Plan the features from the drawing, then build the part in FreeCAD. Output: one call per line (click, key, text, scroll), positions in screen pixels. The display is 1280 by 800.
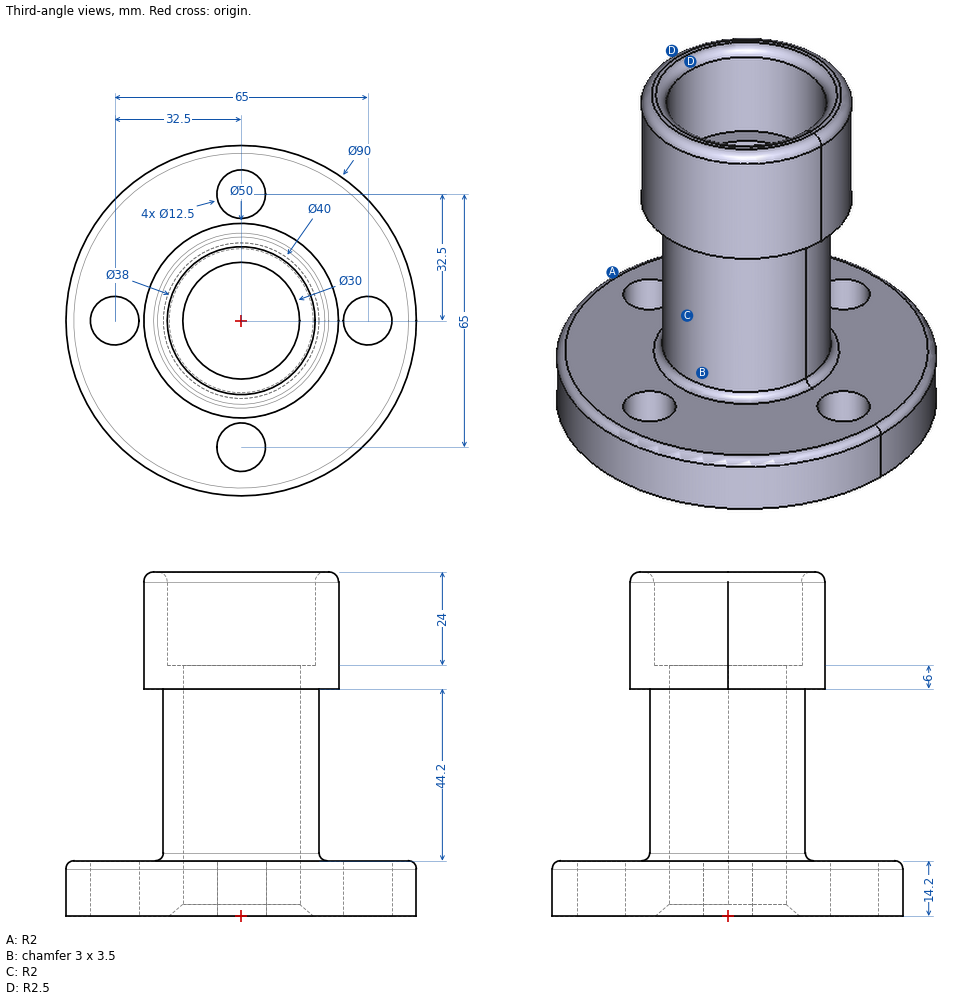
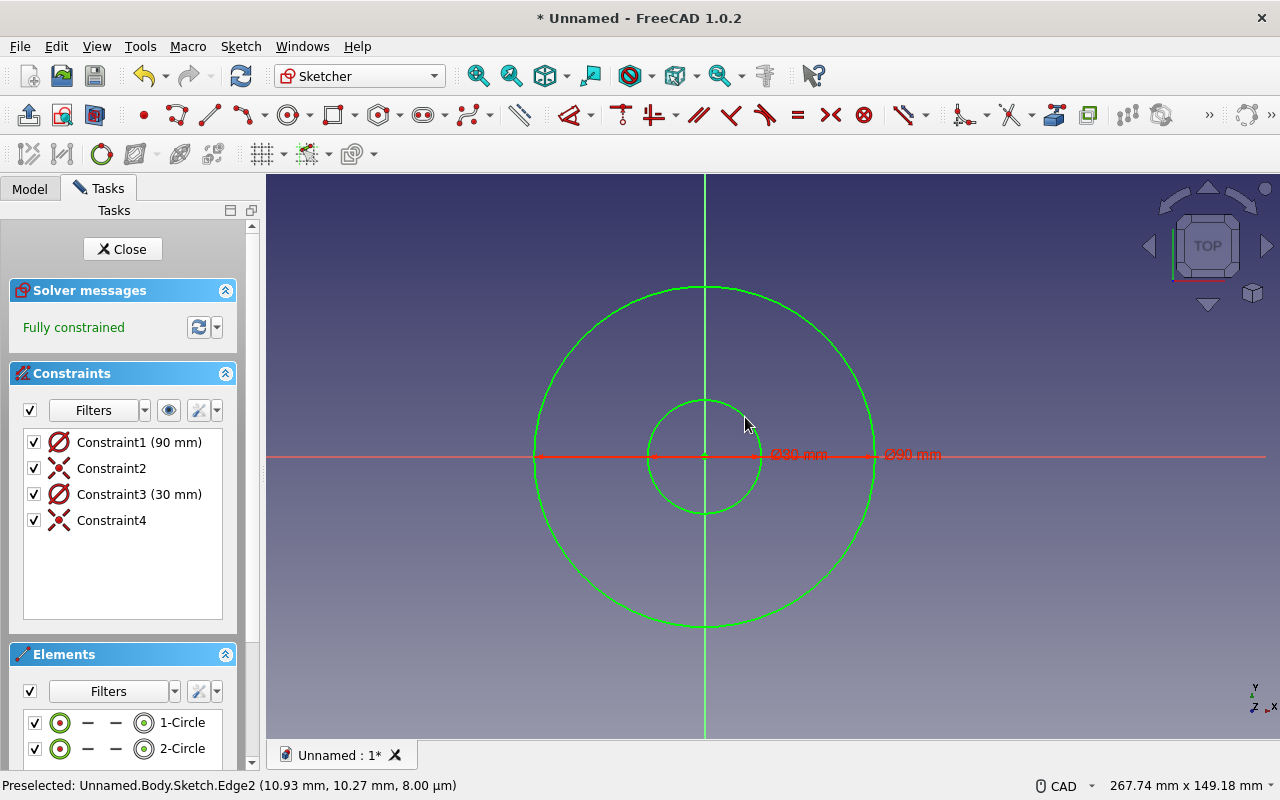
click(123, 249)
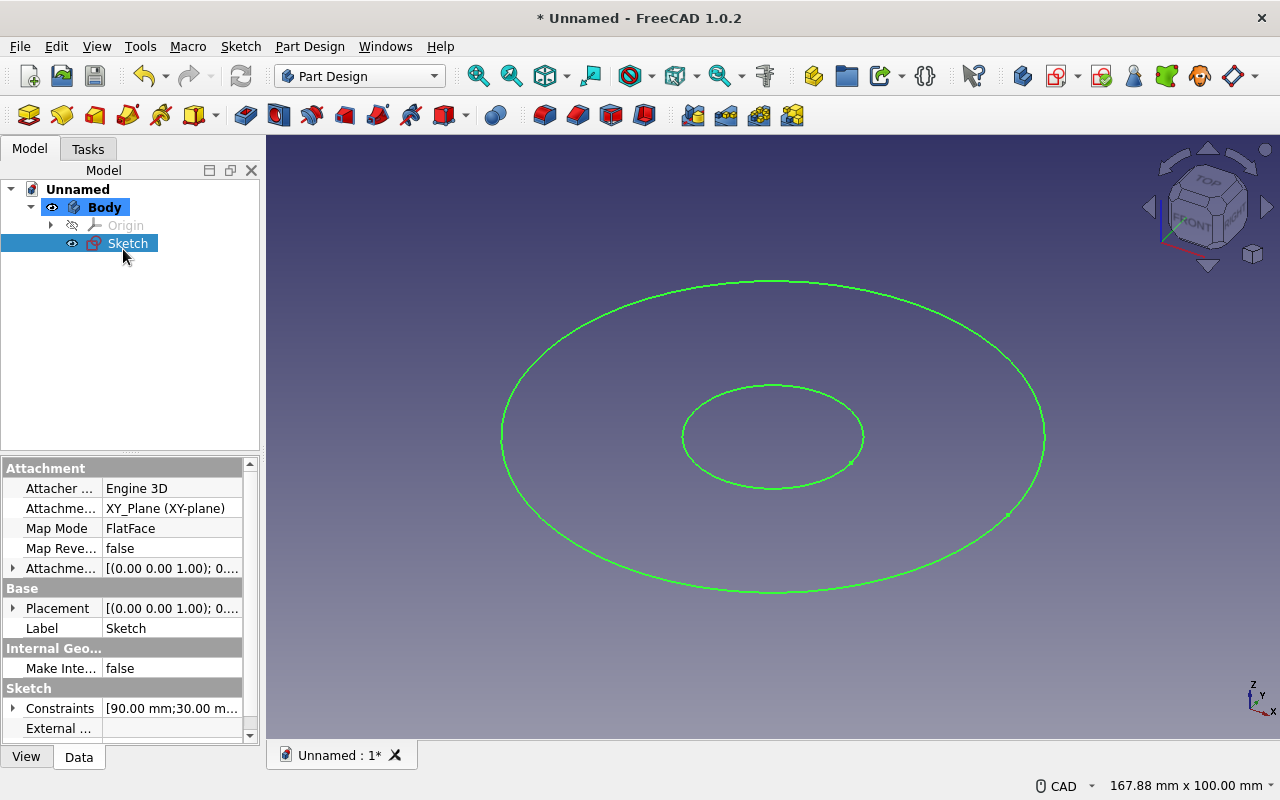
click(29, 116)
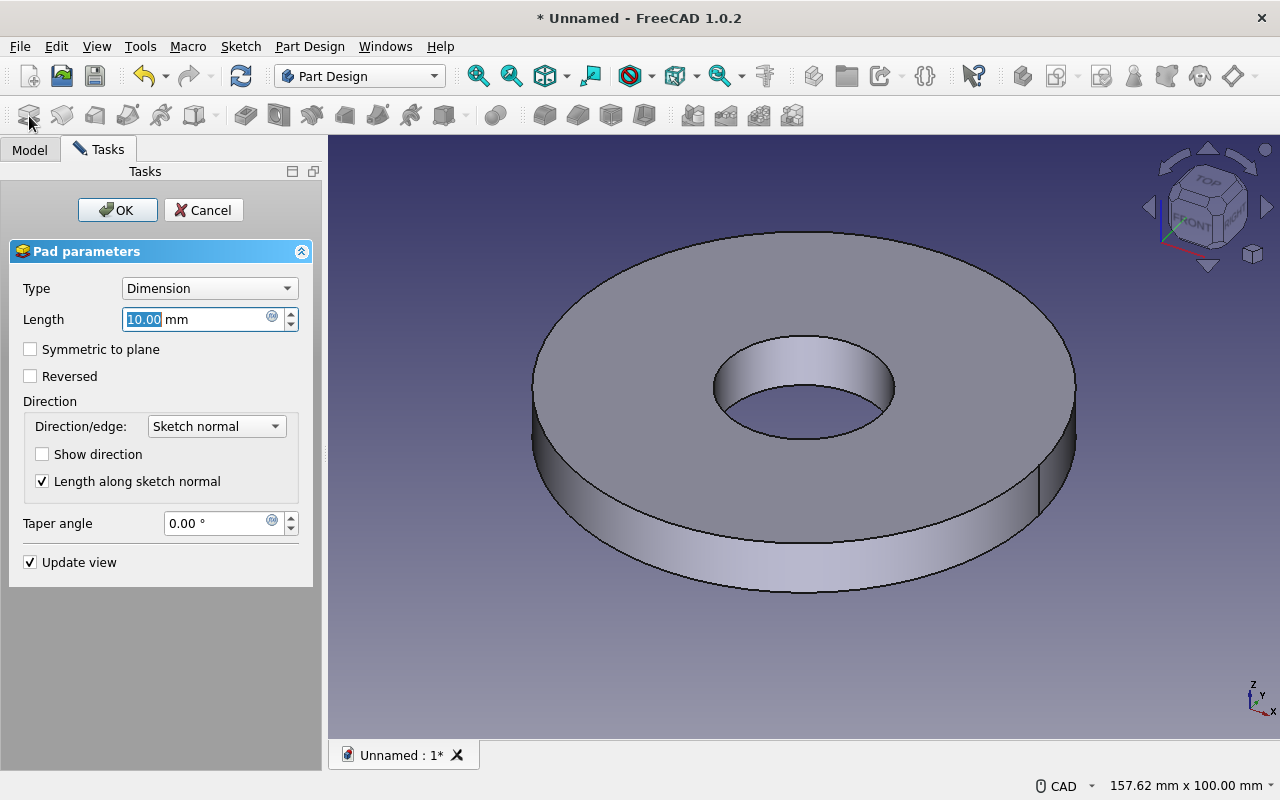
text(14.2)
key(Tab)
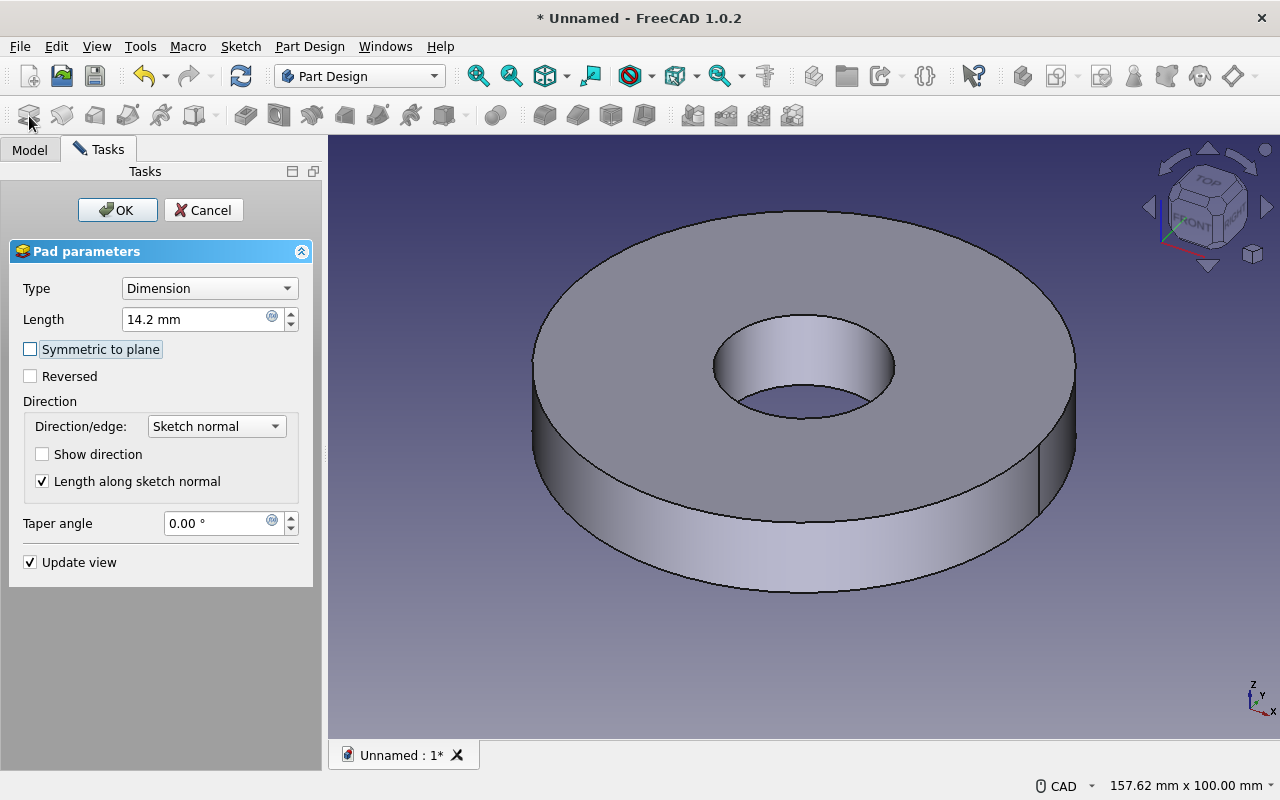
click(118, 210)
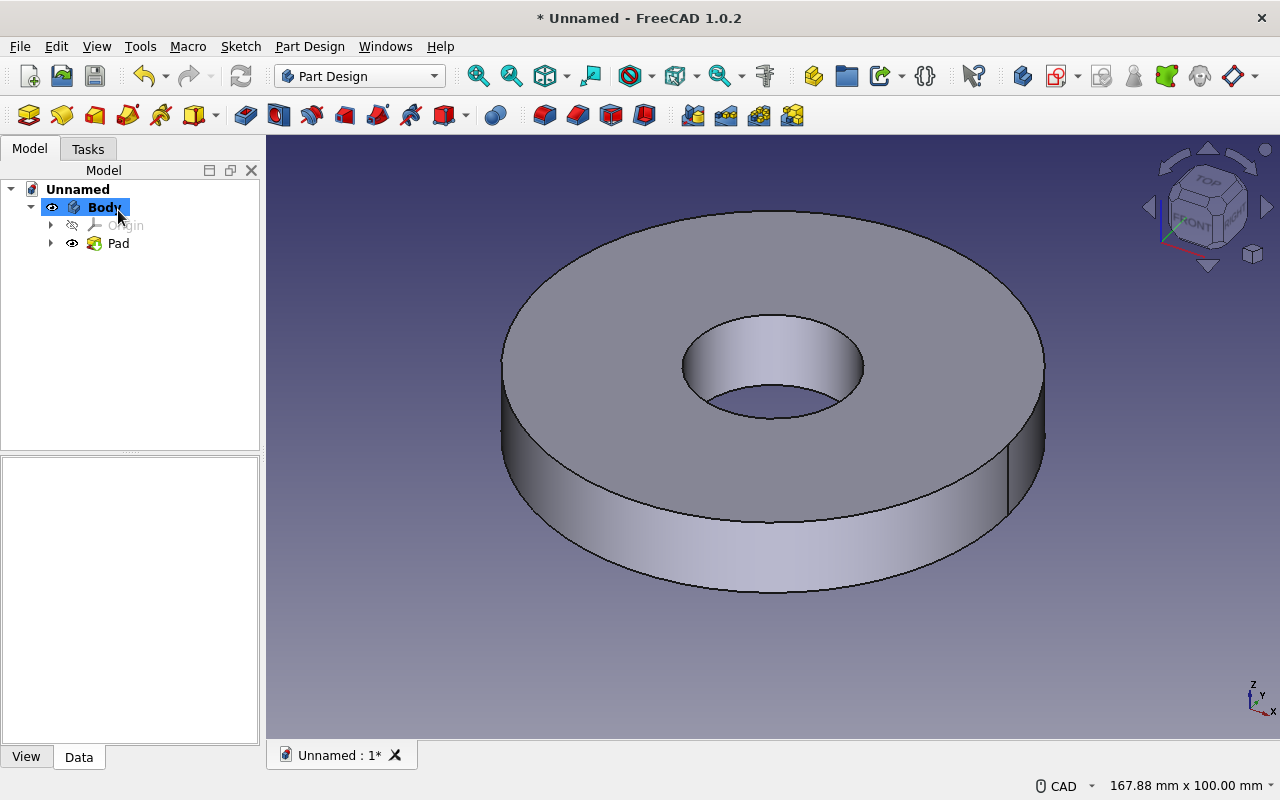
click(628, 421)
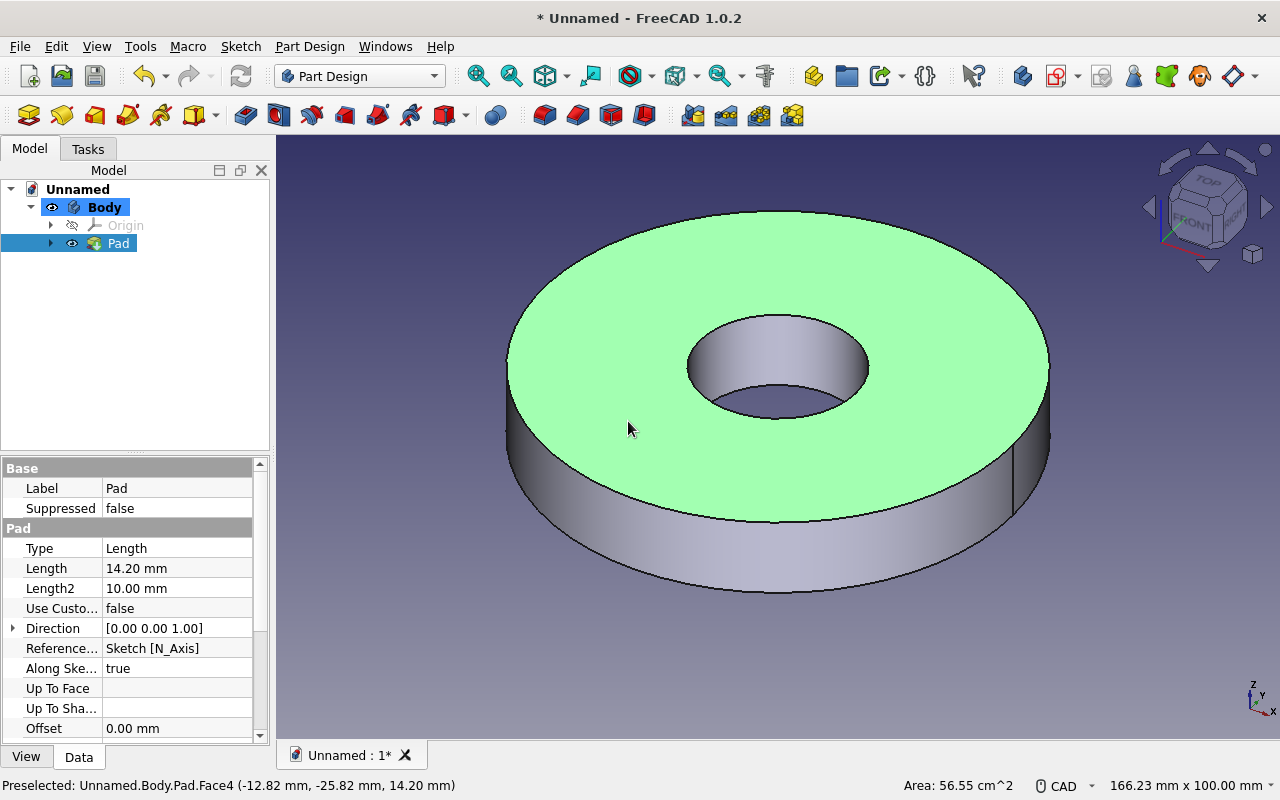
click(1056, 76)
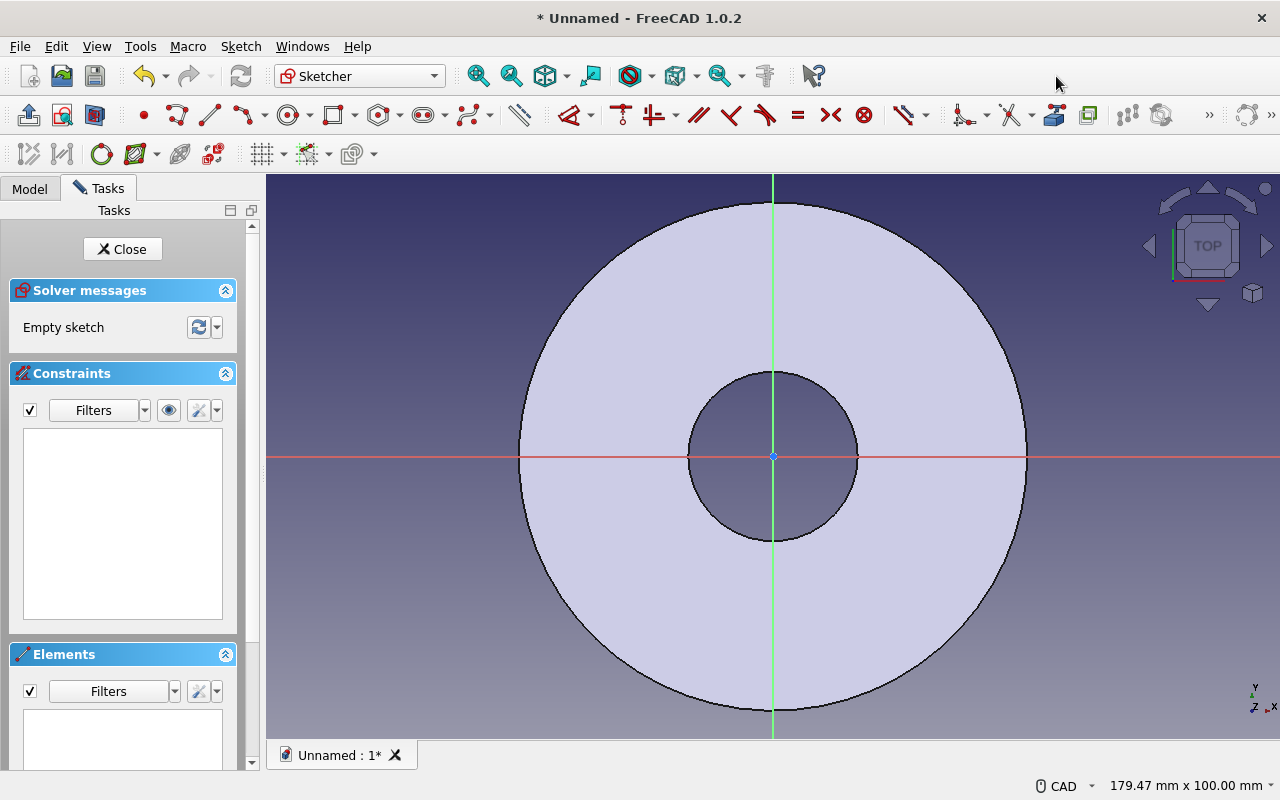
key(g)
key(c)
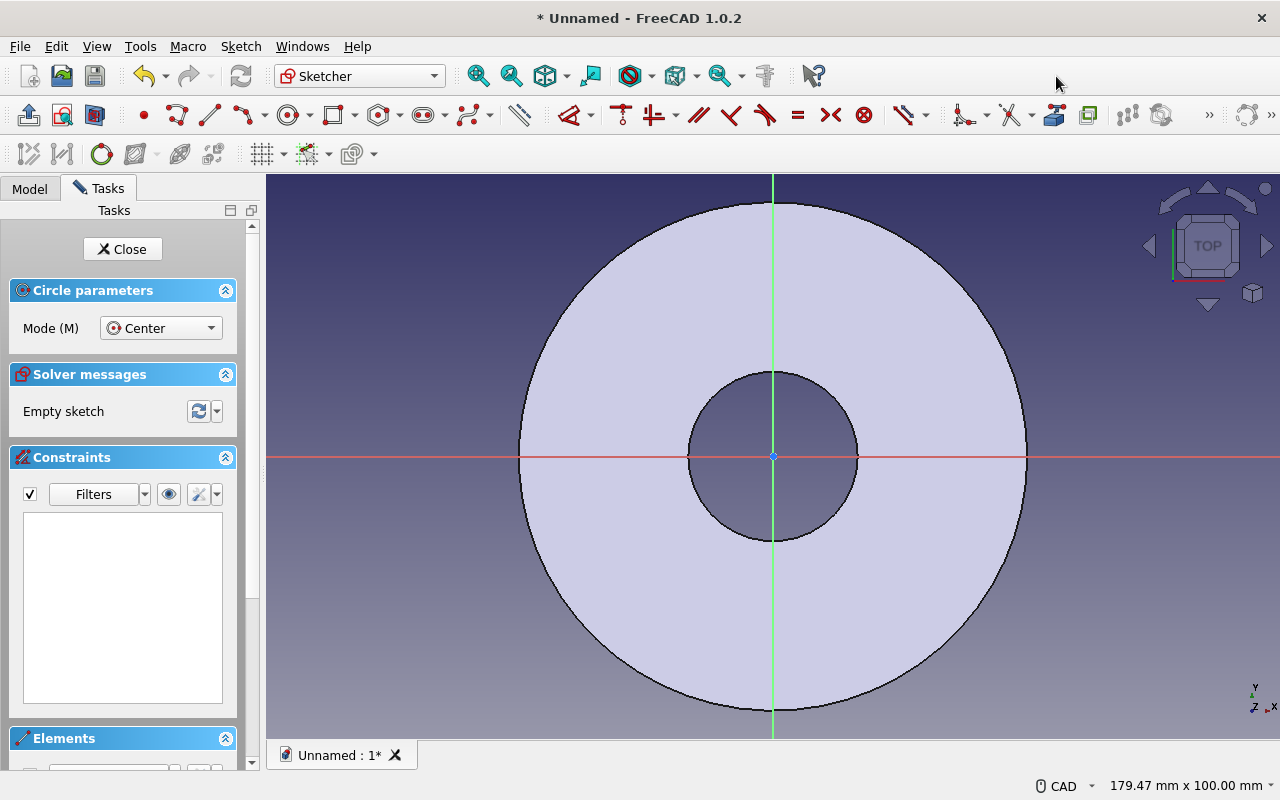
click(773, 273)
move(798, 248)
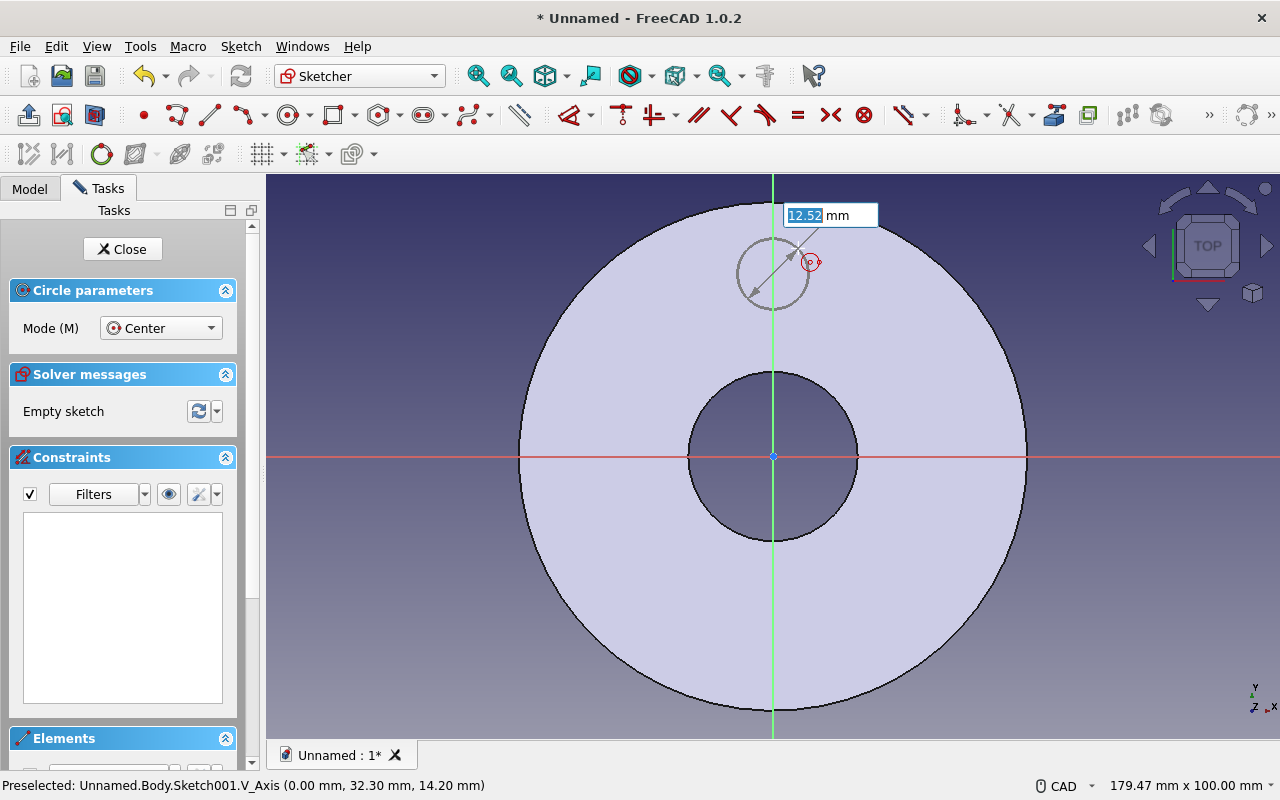
text(12.5)
key(Return)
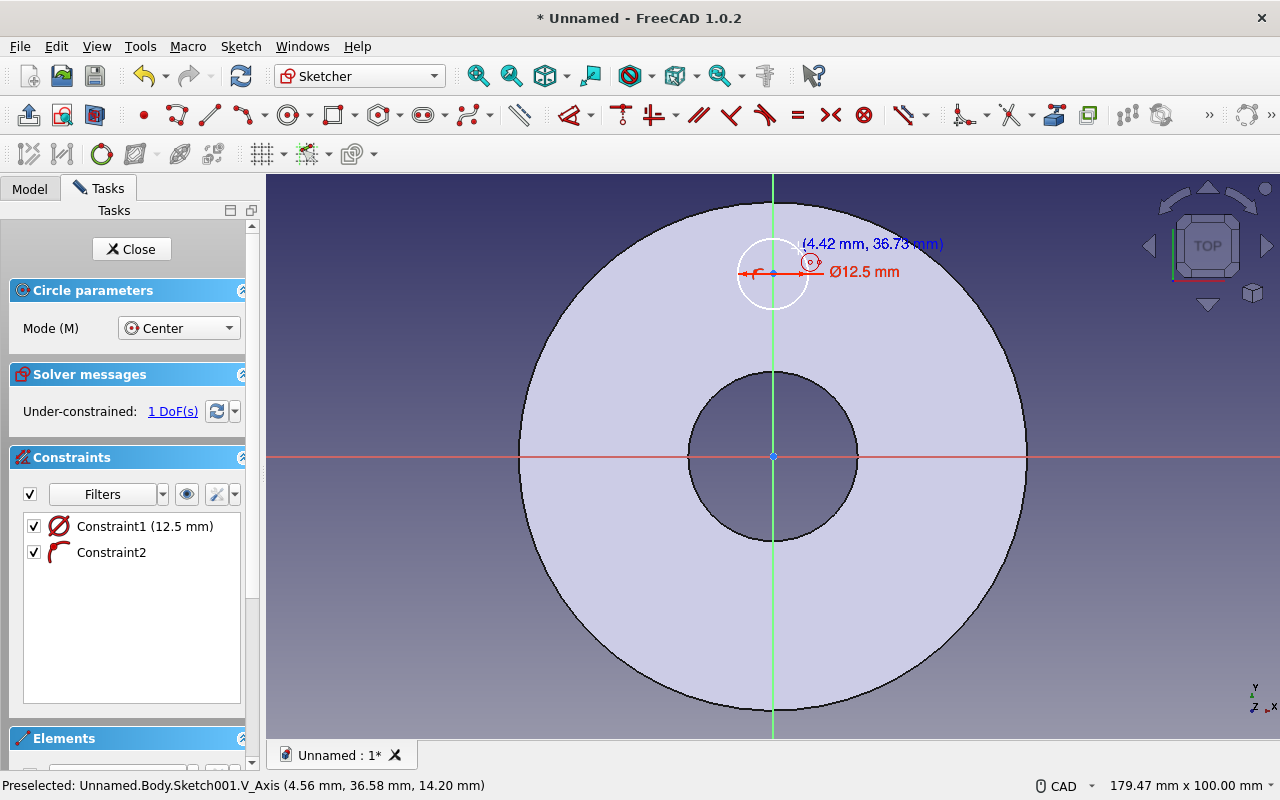
click(589, 456)
move(614, 432)